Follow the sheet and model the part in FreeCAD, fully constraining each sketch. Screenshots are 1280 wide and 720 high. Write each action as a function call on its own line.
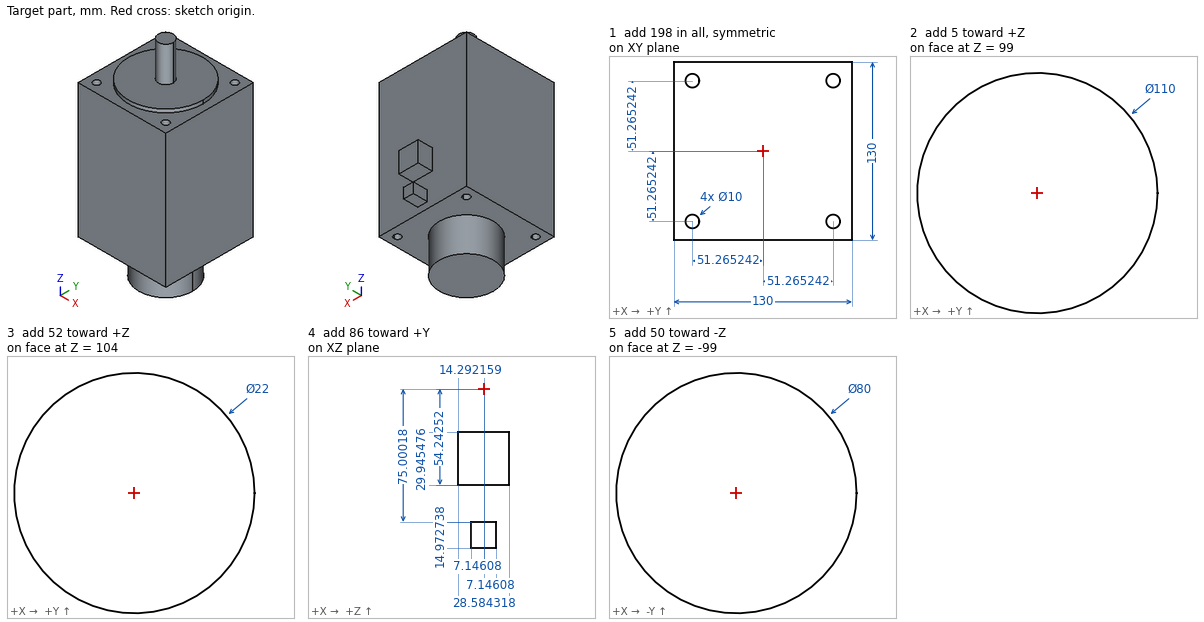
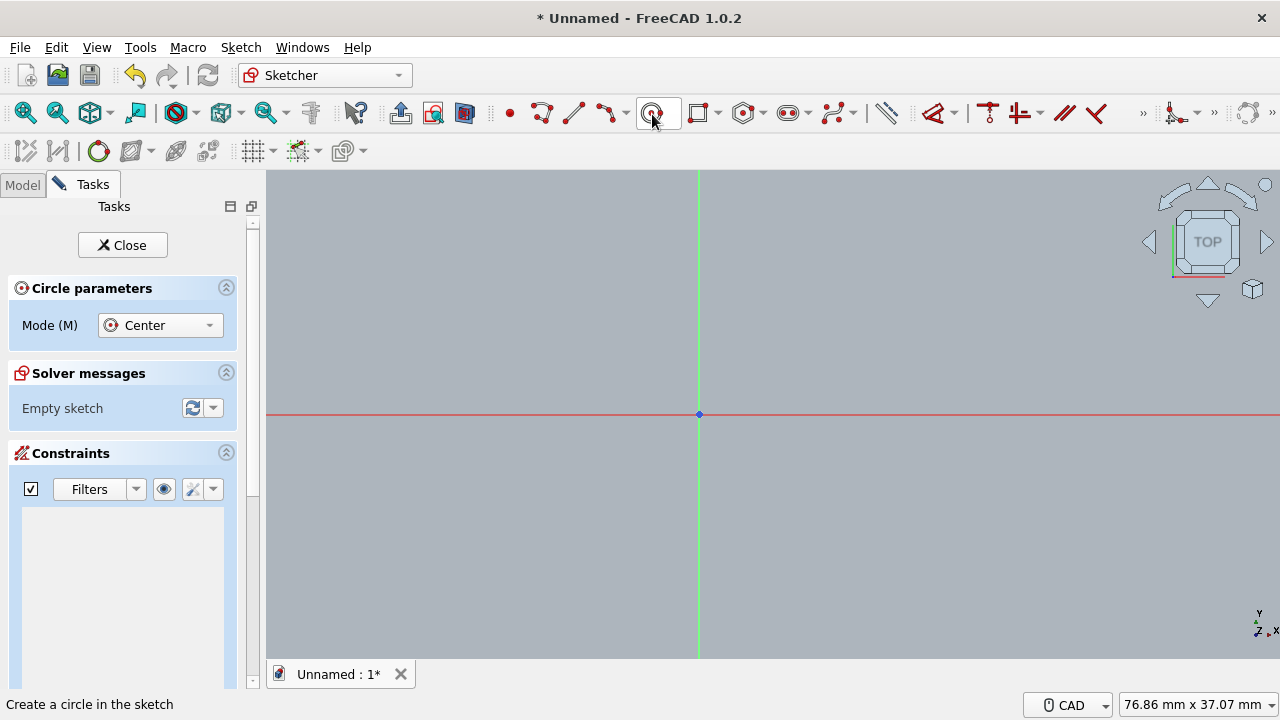
click(699, 414)
click(802, 312)
key(Escape)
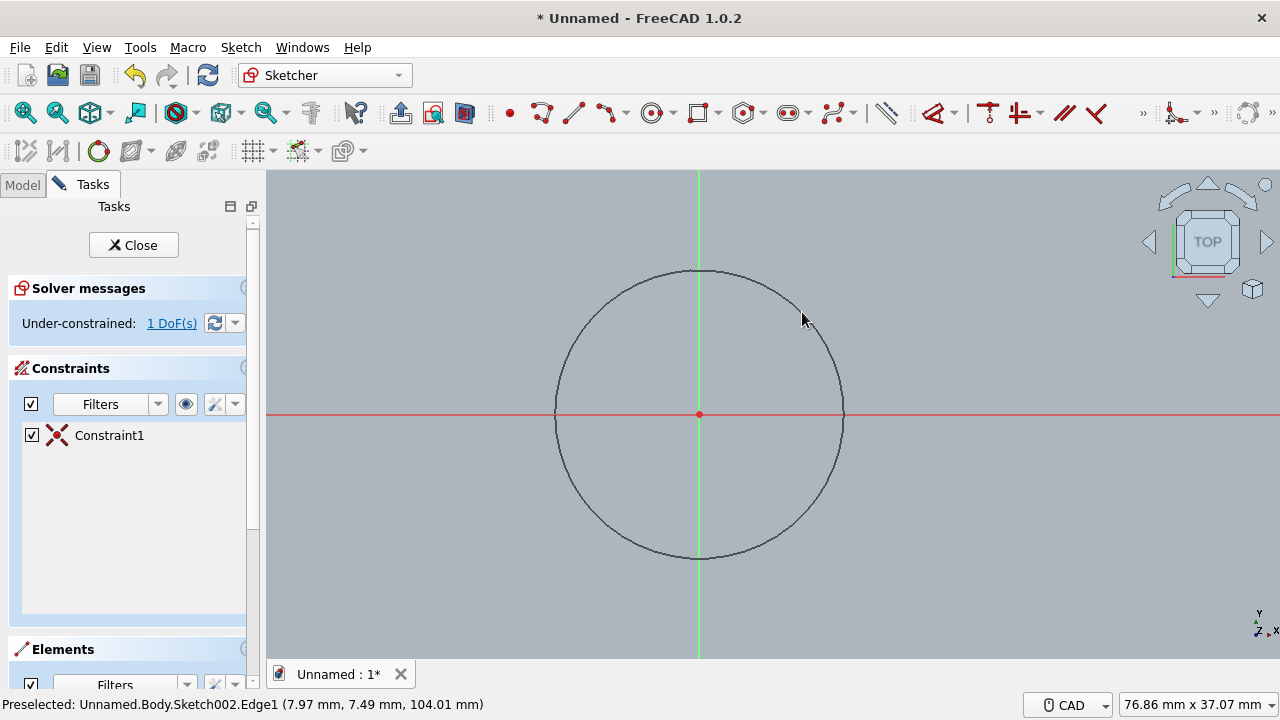
key(d)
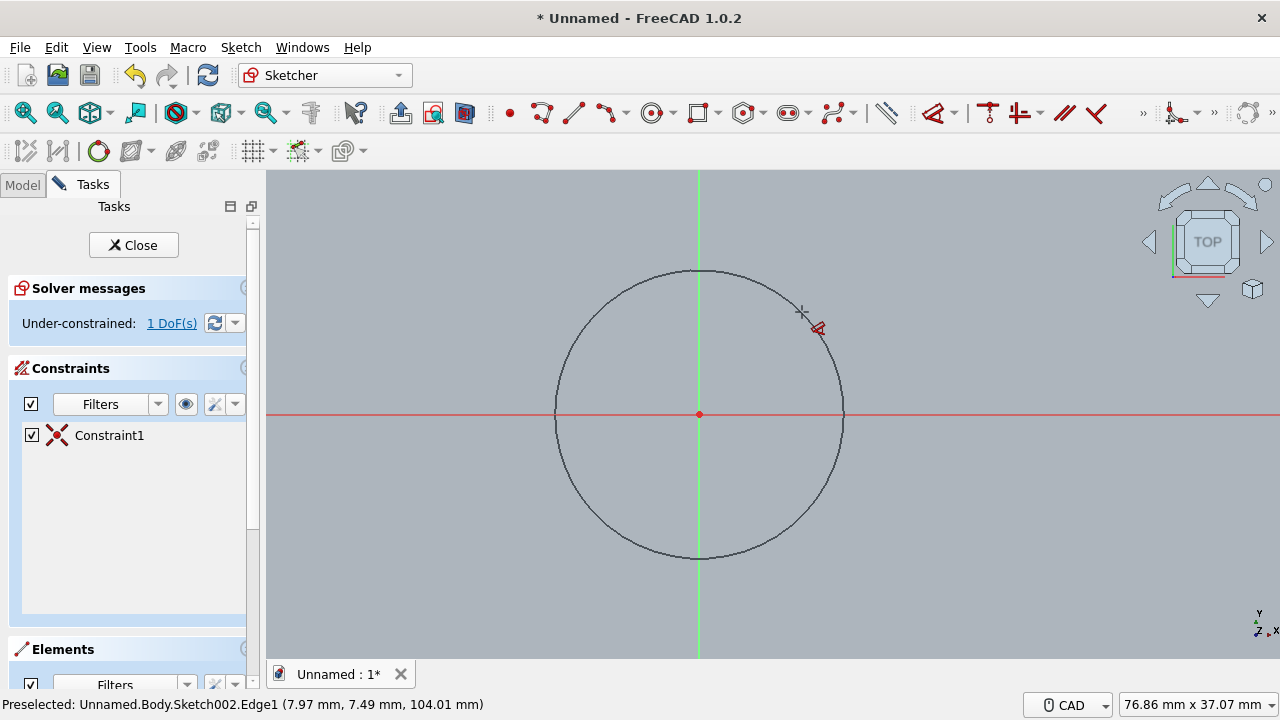
click(801, 312)
click(824, 289)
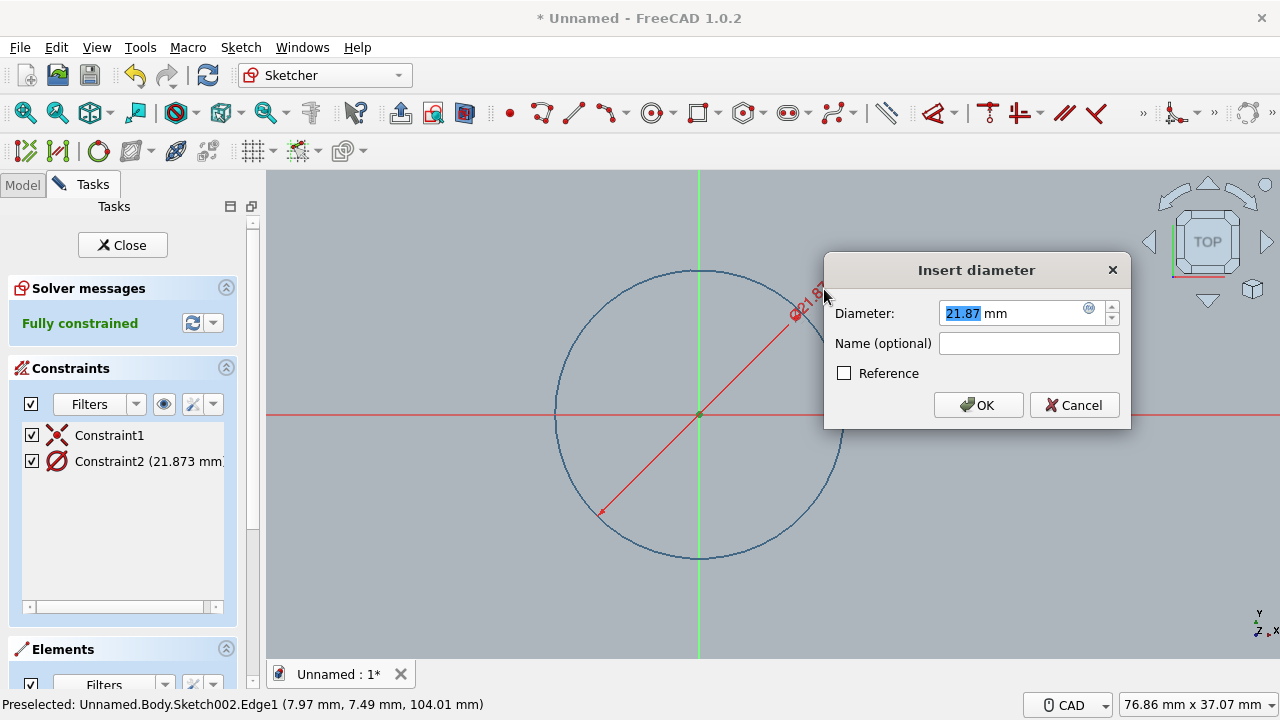
text(22)
key(Return)
key(Escape)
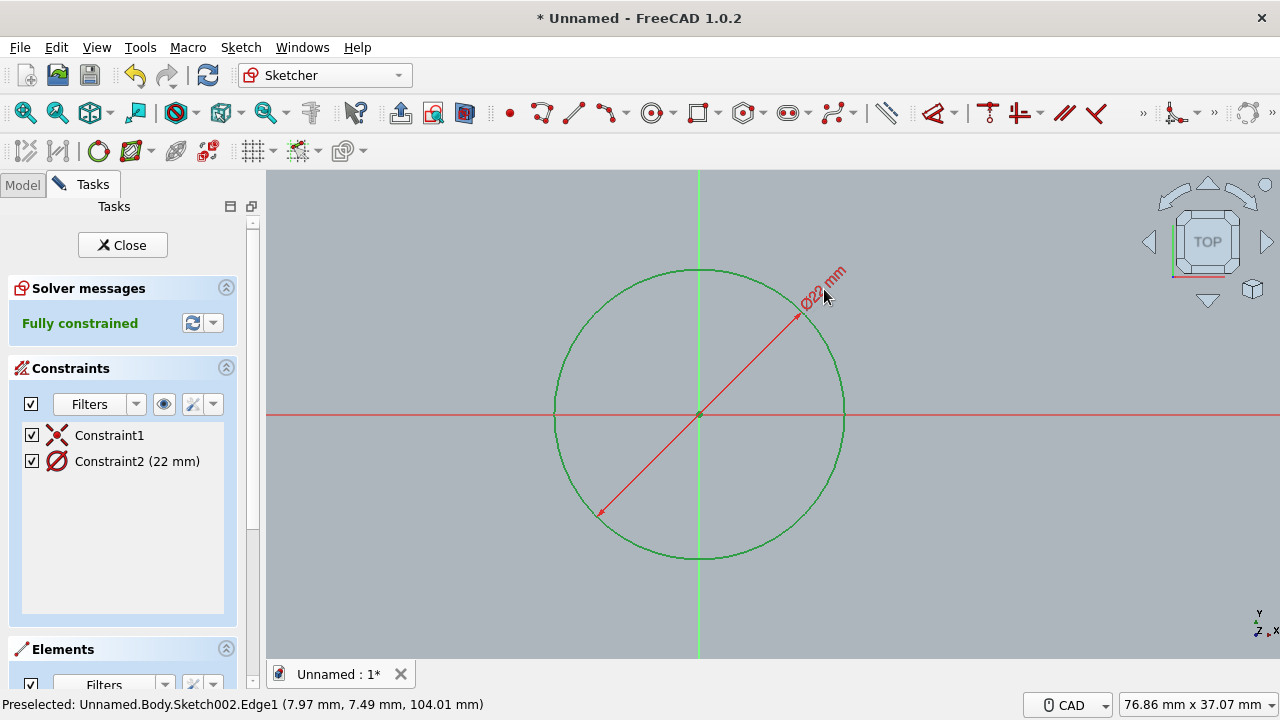
click(123, 245)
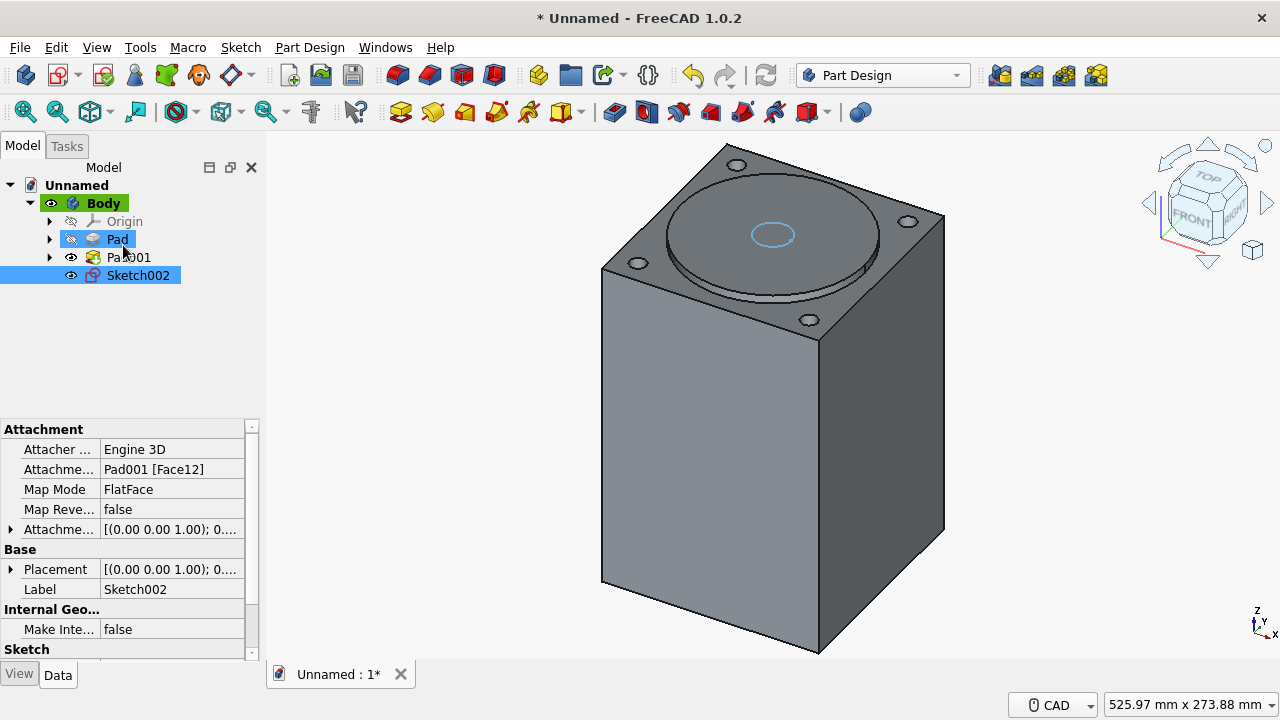
click(402, 112)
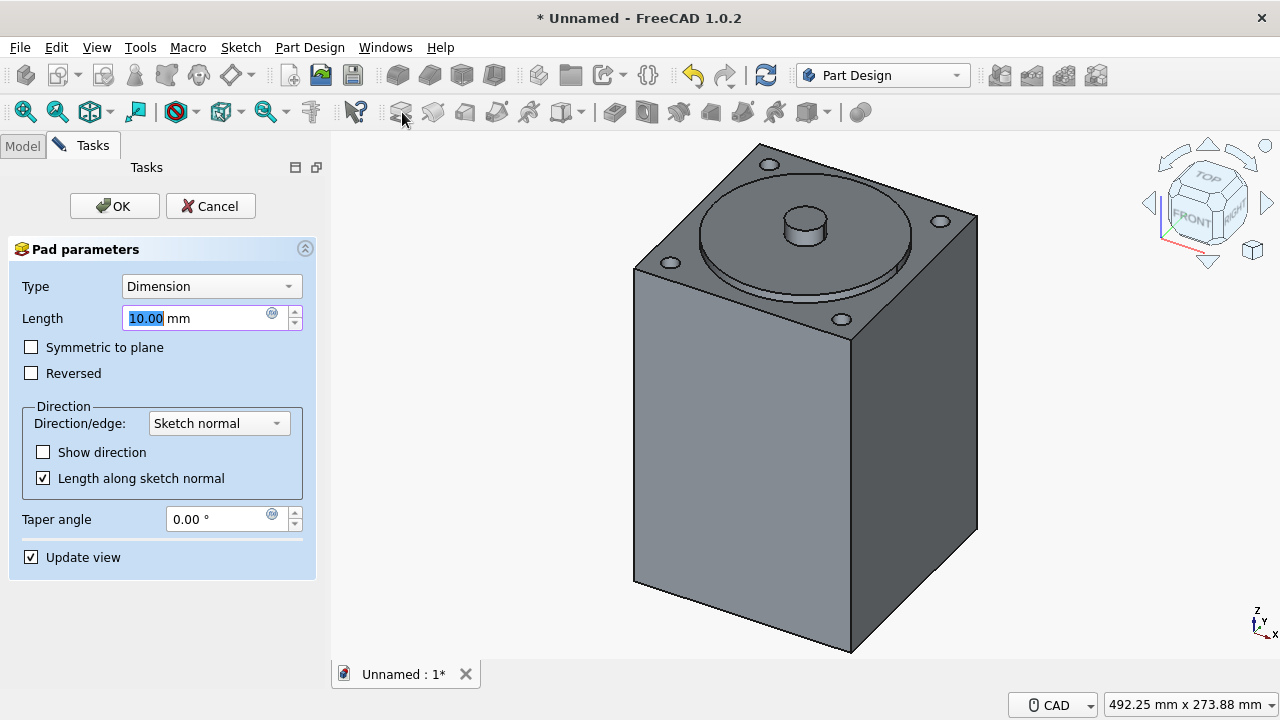
text(52)
key(Tab)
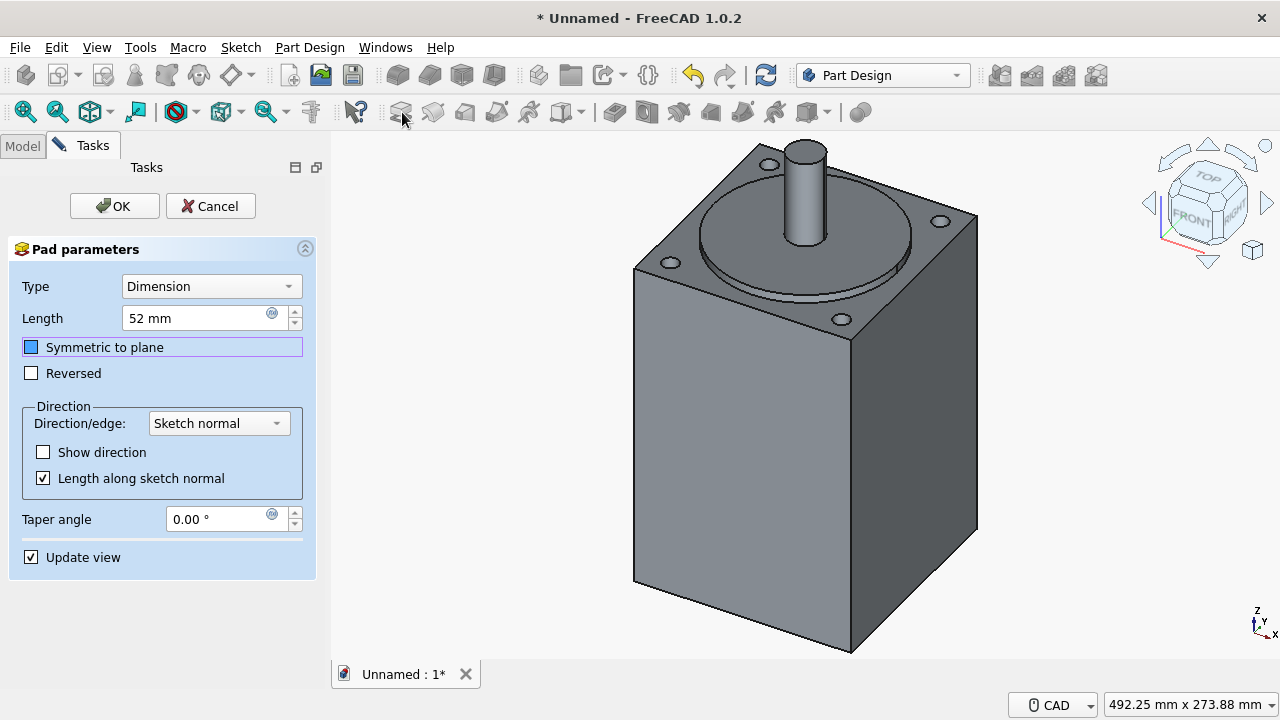
click(115, 206)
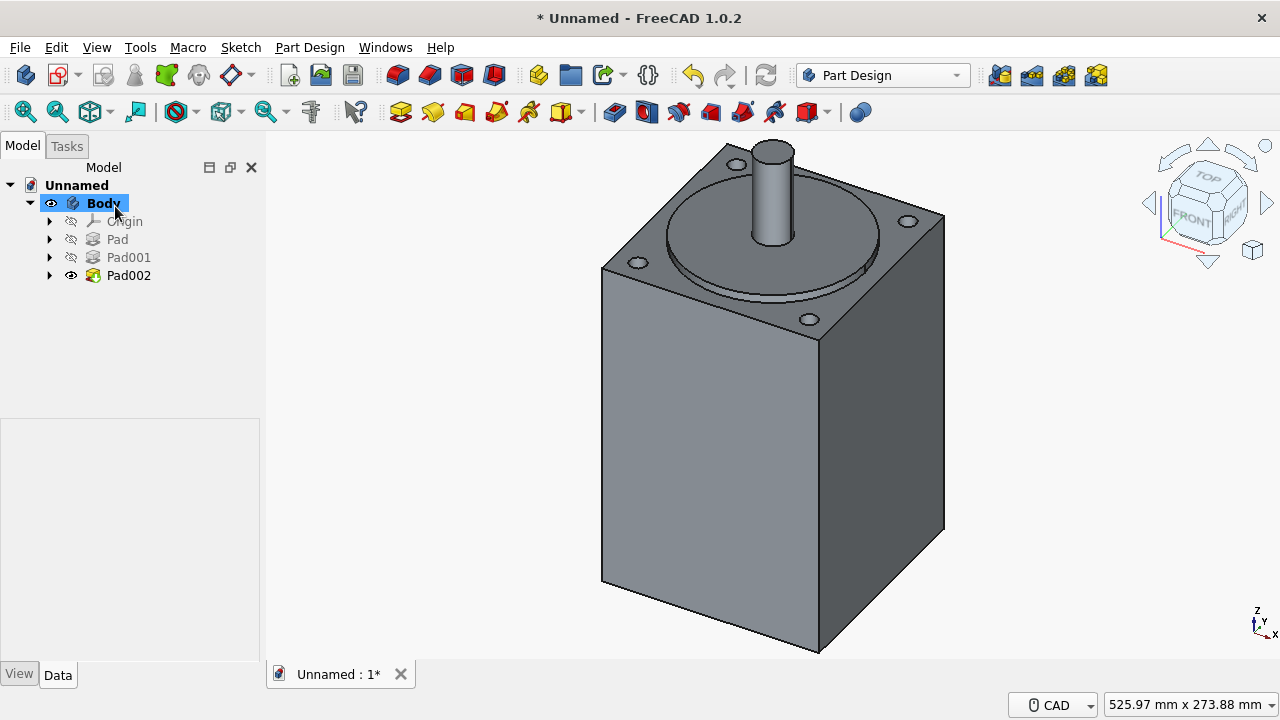
key(v)
key(f)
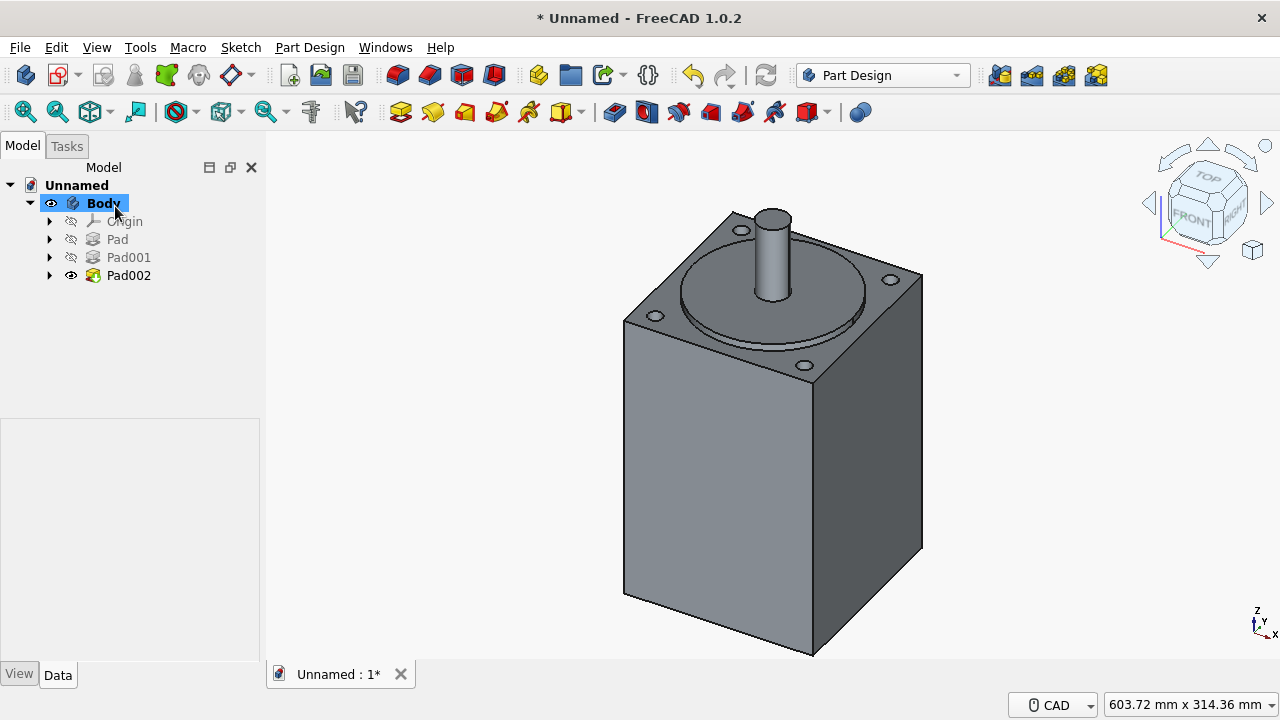
click(58, 76)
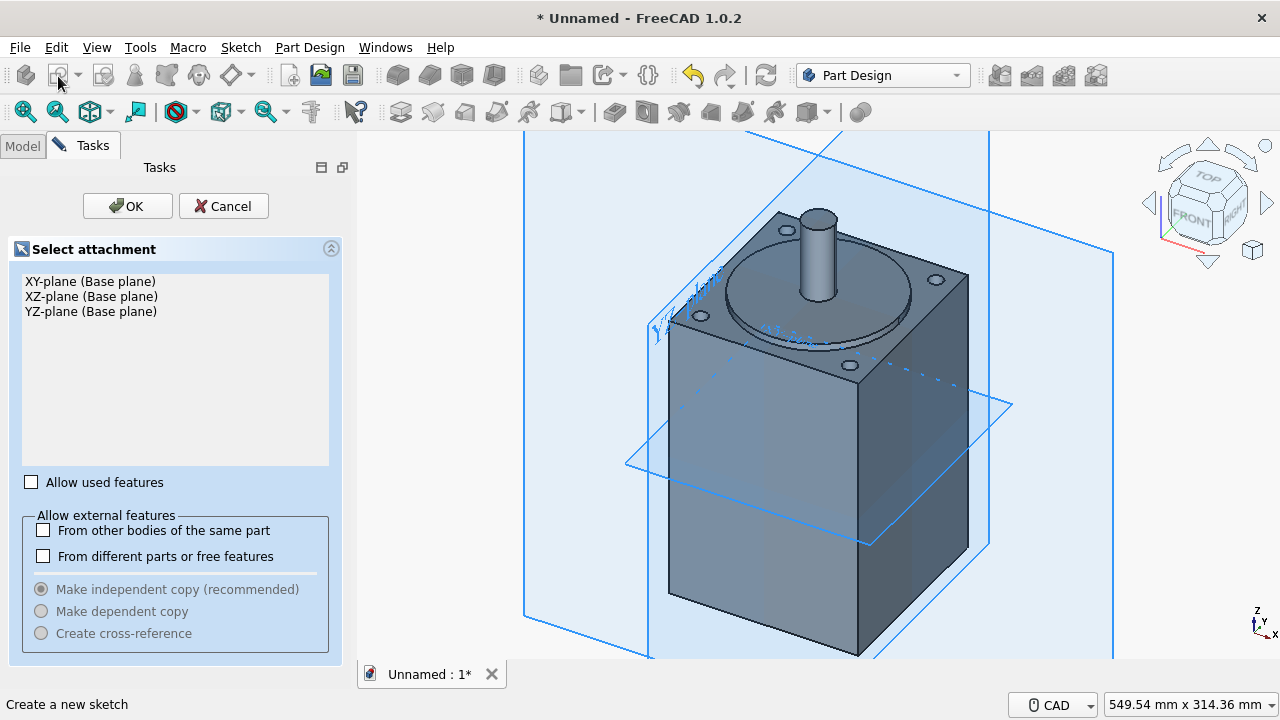
click(82, 296)